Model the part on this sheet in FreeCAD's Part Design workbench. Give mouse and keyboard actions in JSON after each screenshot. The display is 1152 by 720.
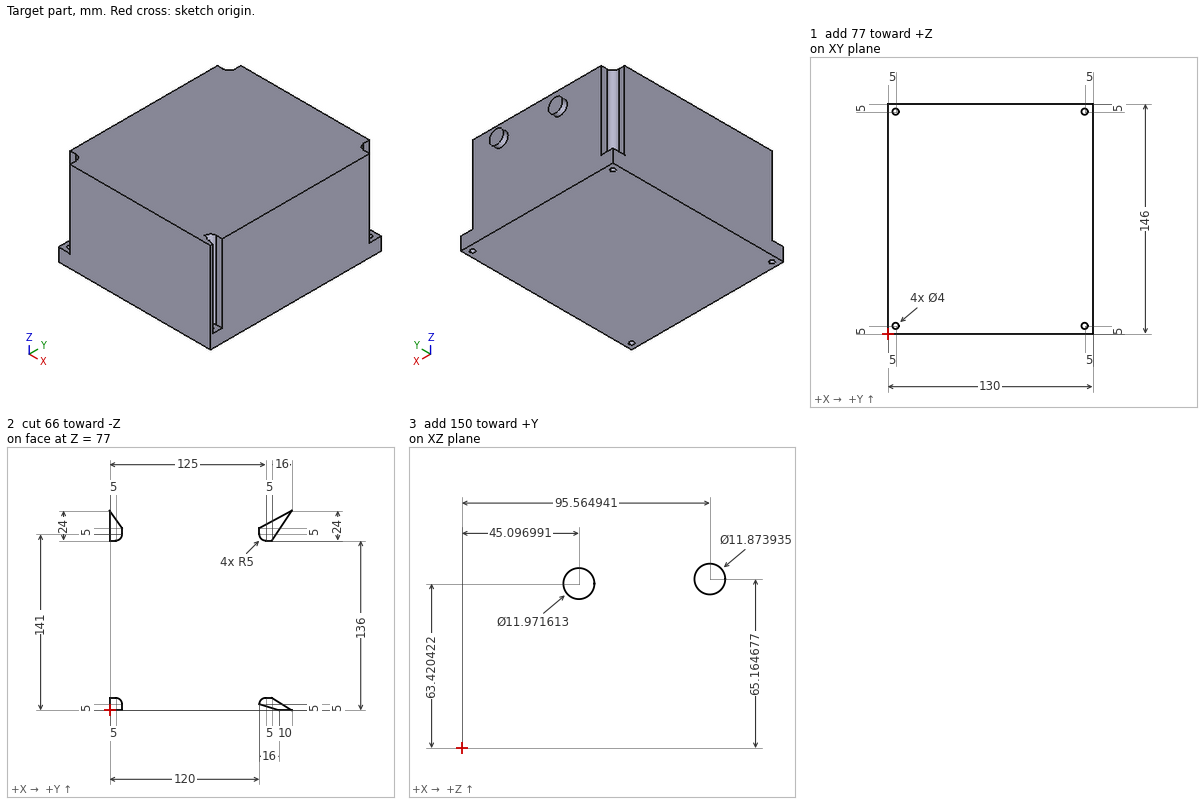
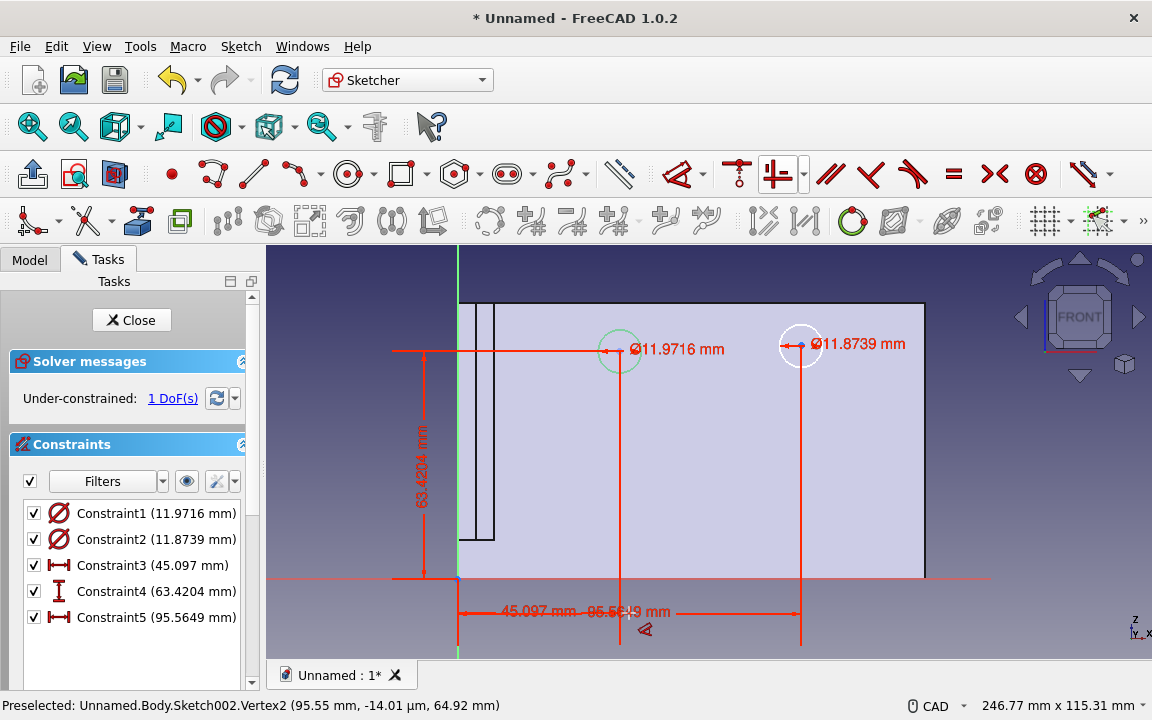
{"action": "left_click", "coordinate": [801, 346]}
{"action": "left_click", "coordinate": [424, 409]}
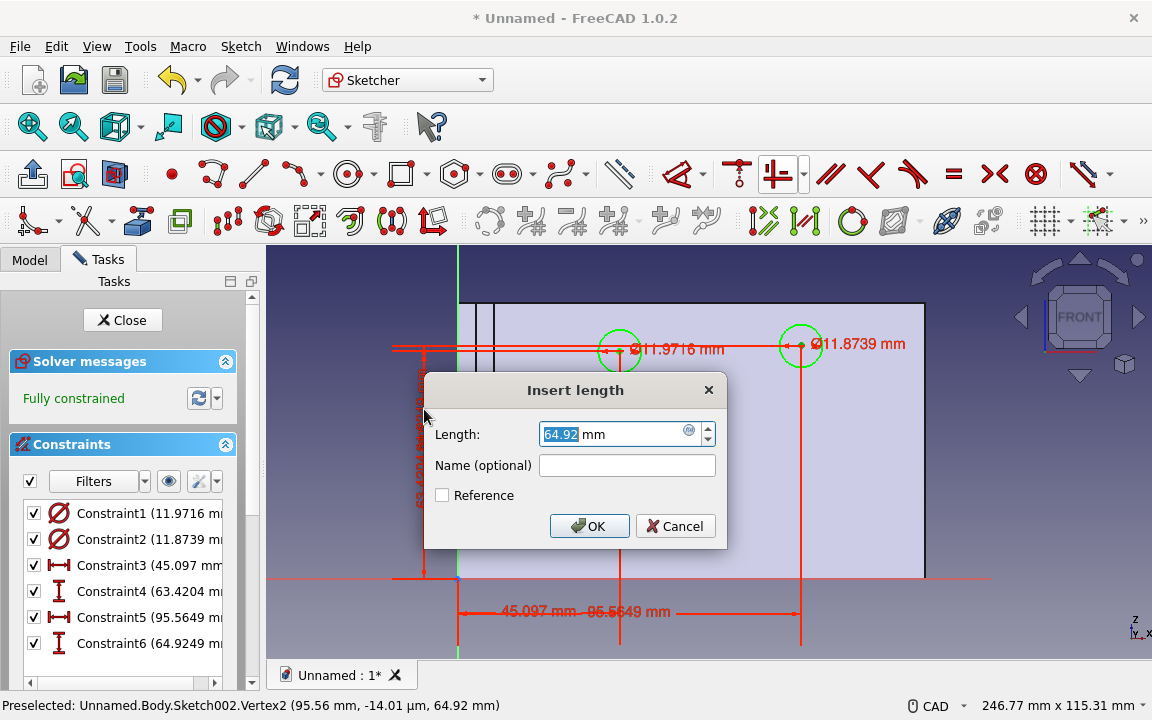
{"action": "type", "text": "65.164677"}
{"action": "key", "text": "Return"}
{"action": "key", "text": "Escape"}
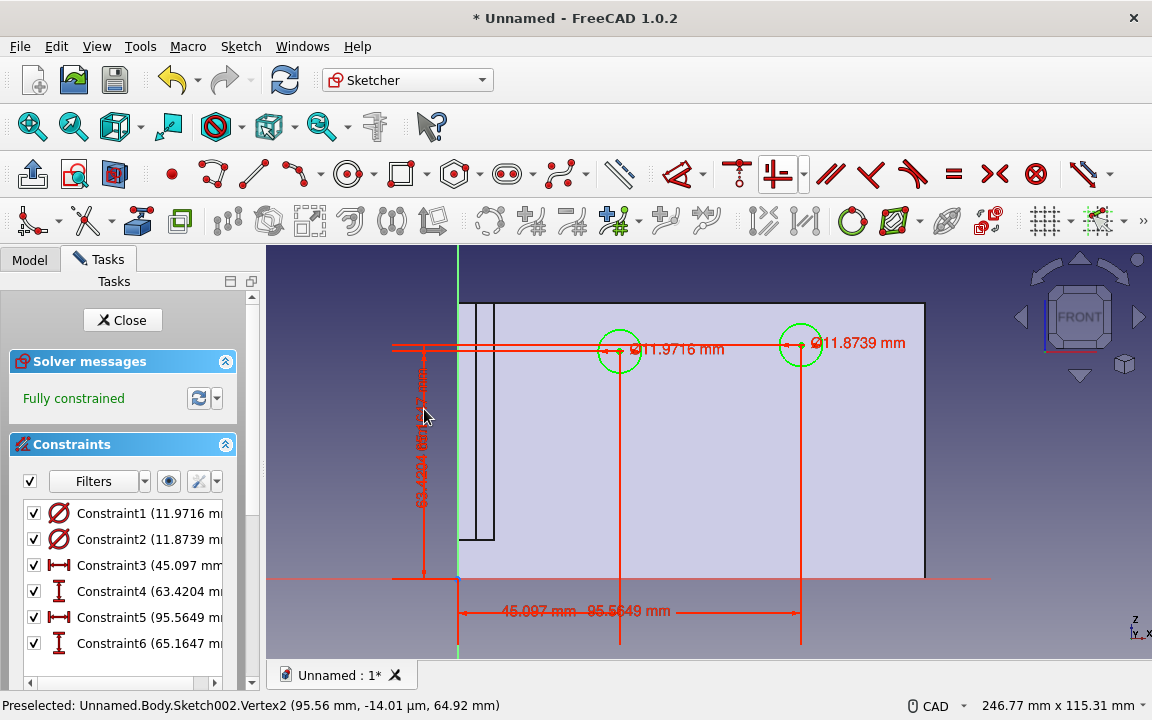
{"action": "left_click", "coordinate": [123, 320]}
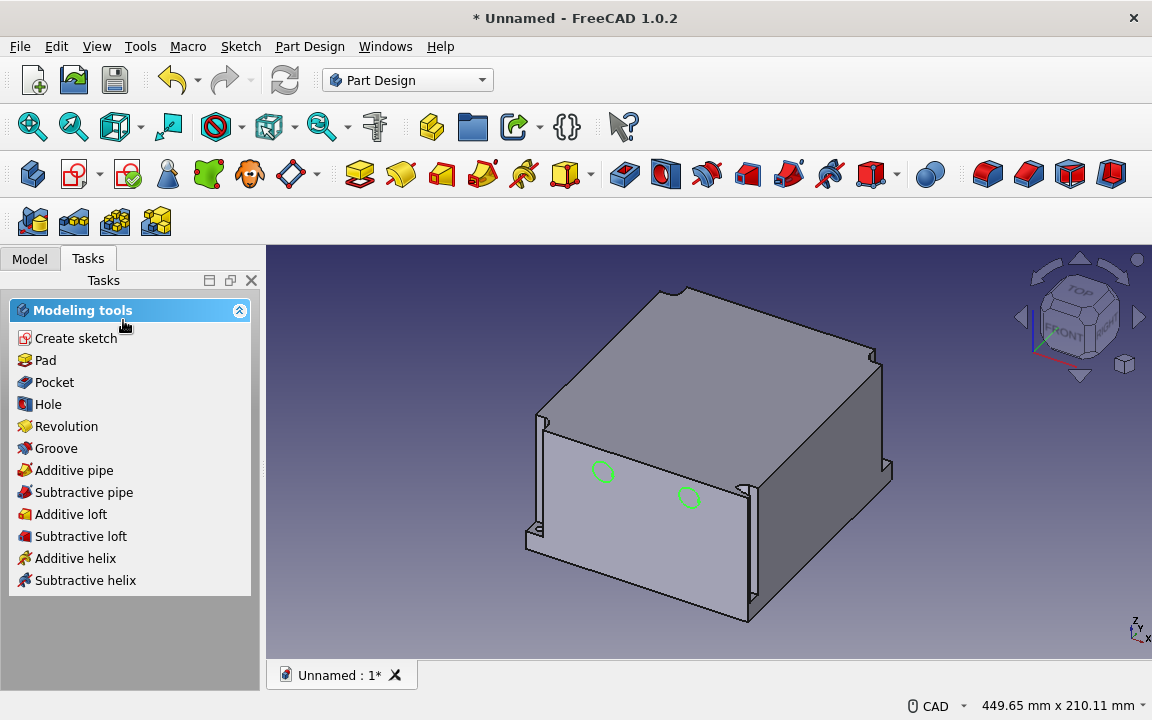
{"action": "left_click", "coordinate": [360, 174]}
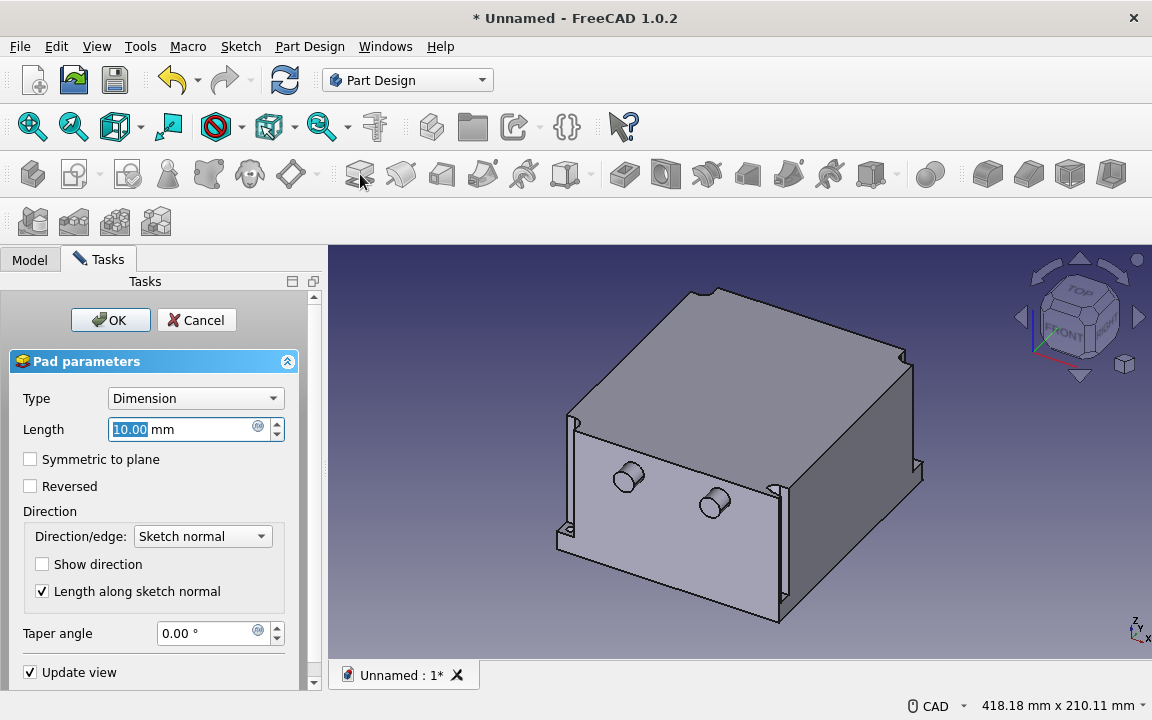
{"action": "type", "text": "150"}
{"action": "key", "text": "Tab"}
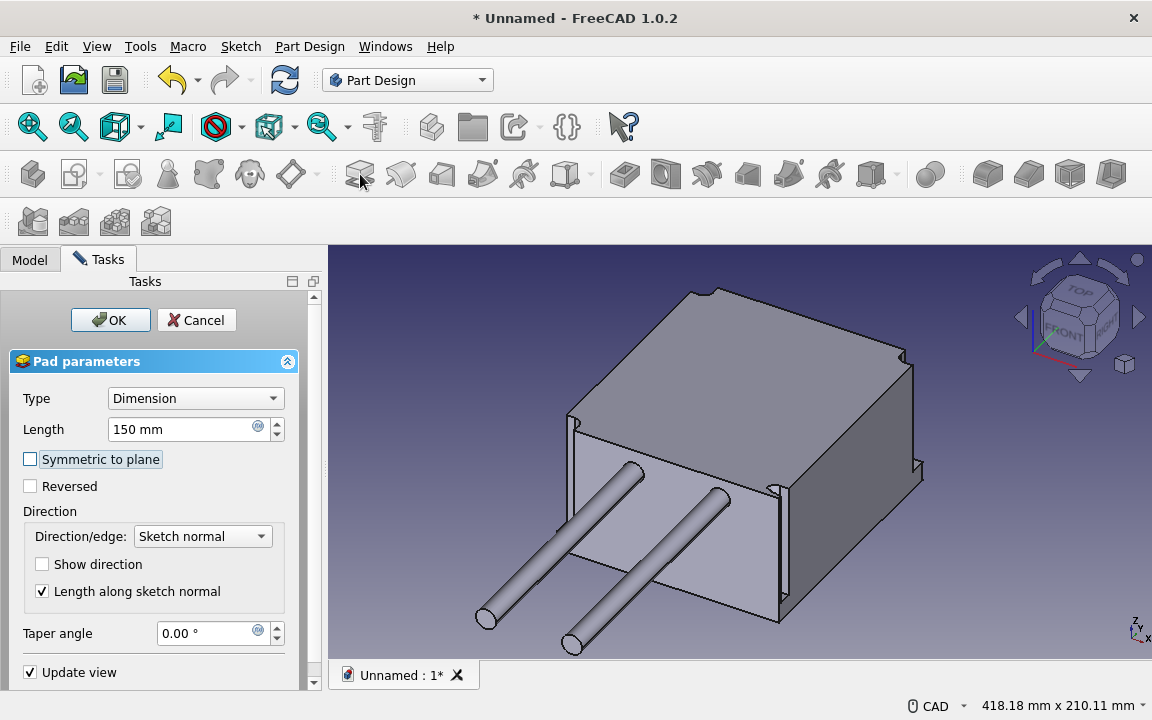
{"action": "left_click", "coordinate": [31, 486]}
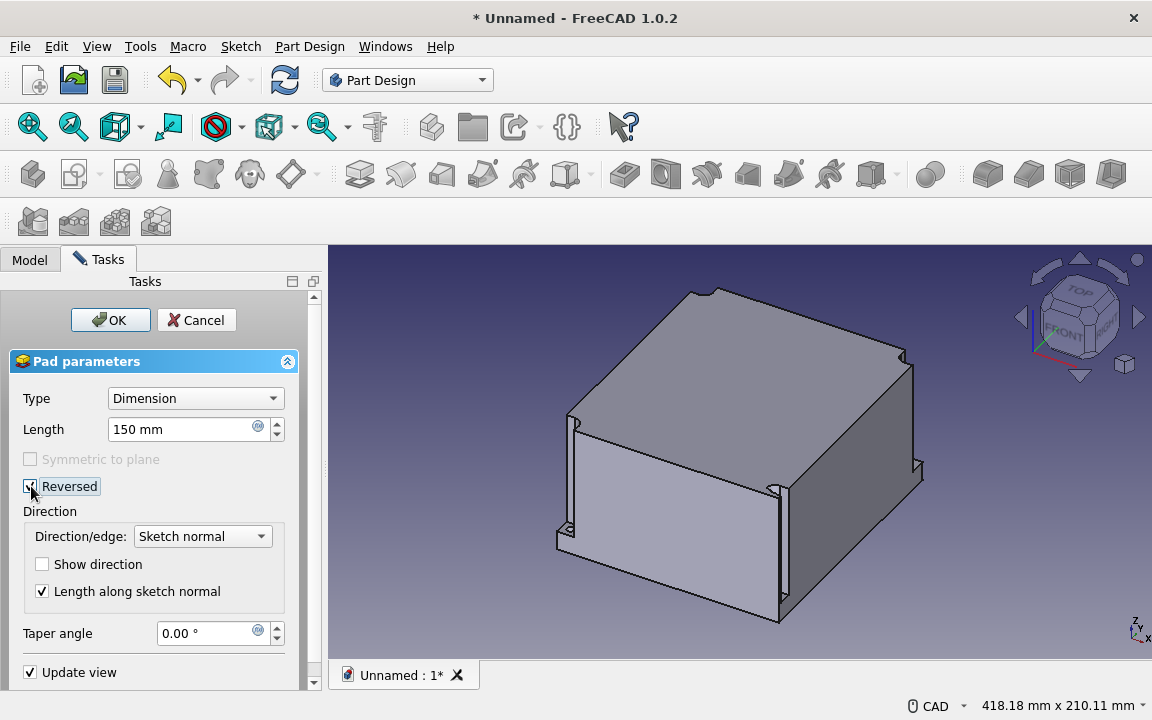
{"action": "left_click", "coordinate": [111, 320]}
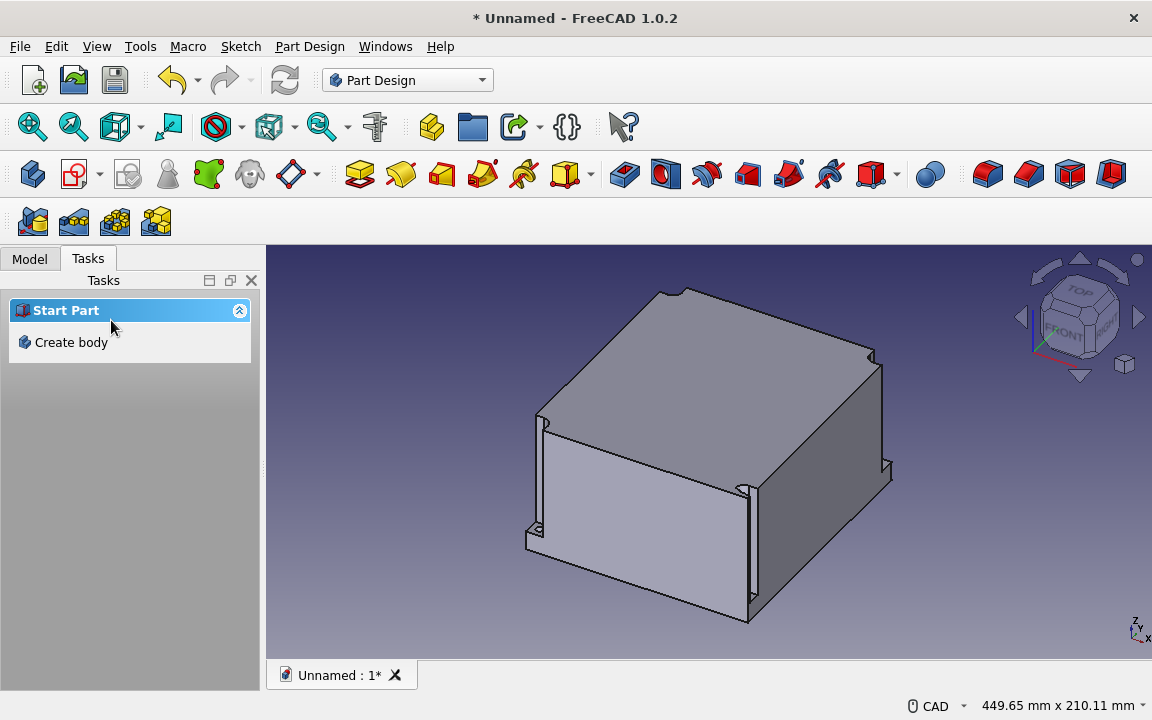
{"action": "key", "text": "0"}